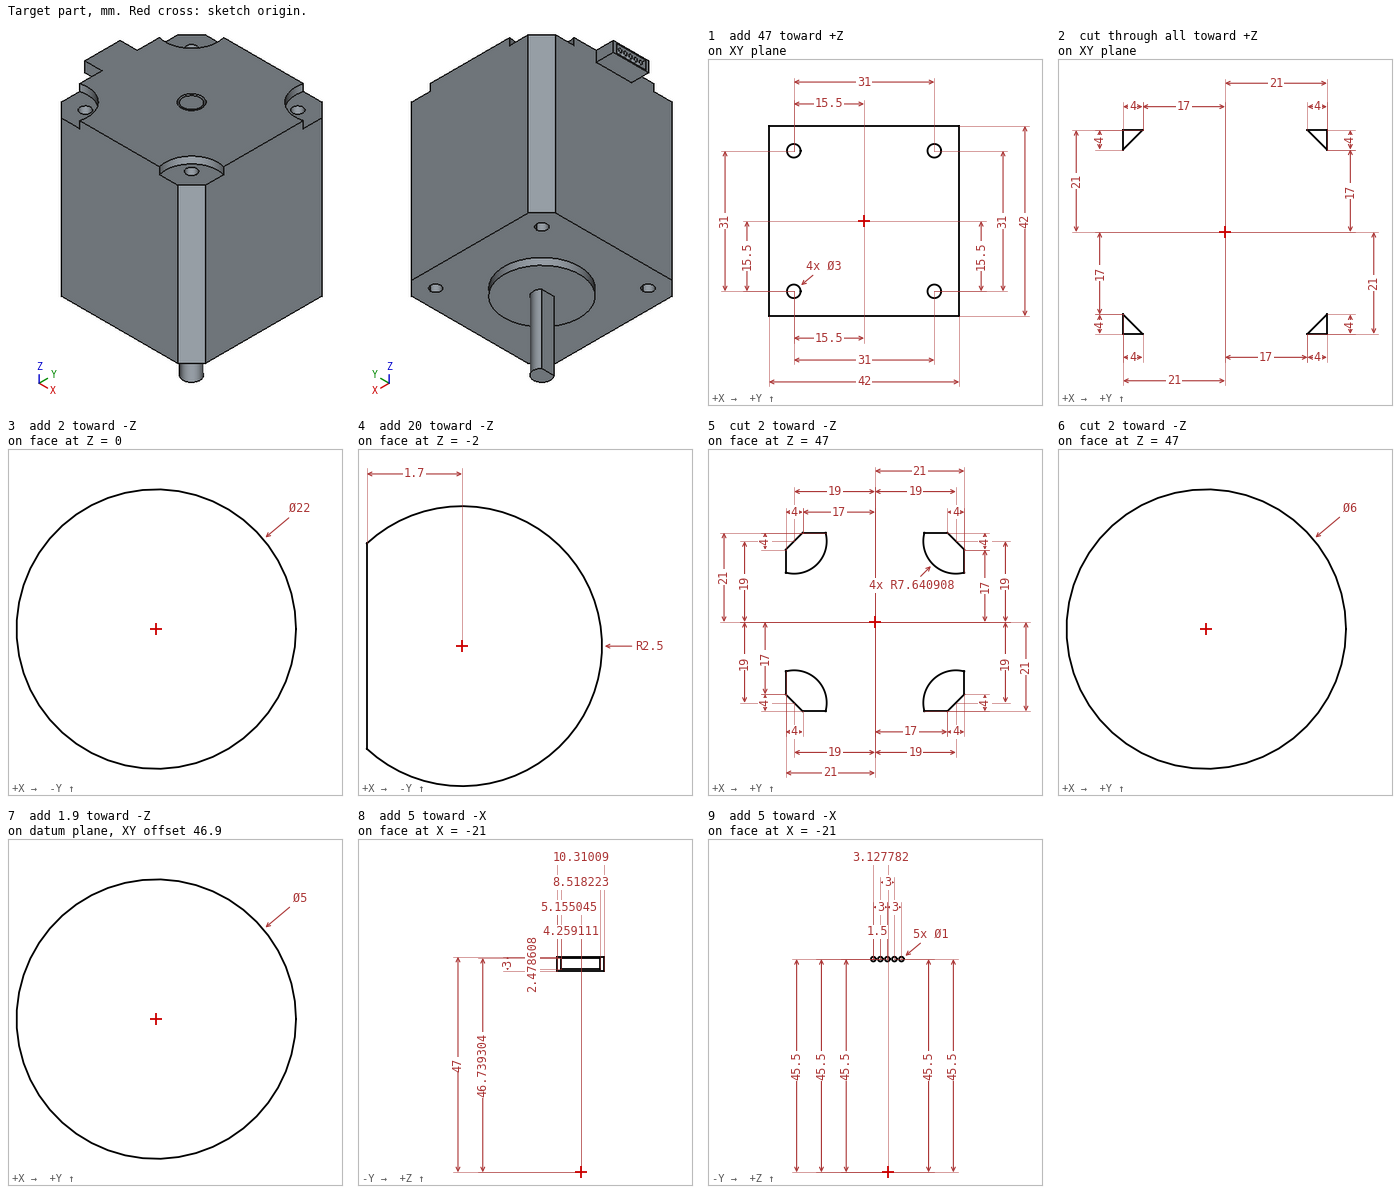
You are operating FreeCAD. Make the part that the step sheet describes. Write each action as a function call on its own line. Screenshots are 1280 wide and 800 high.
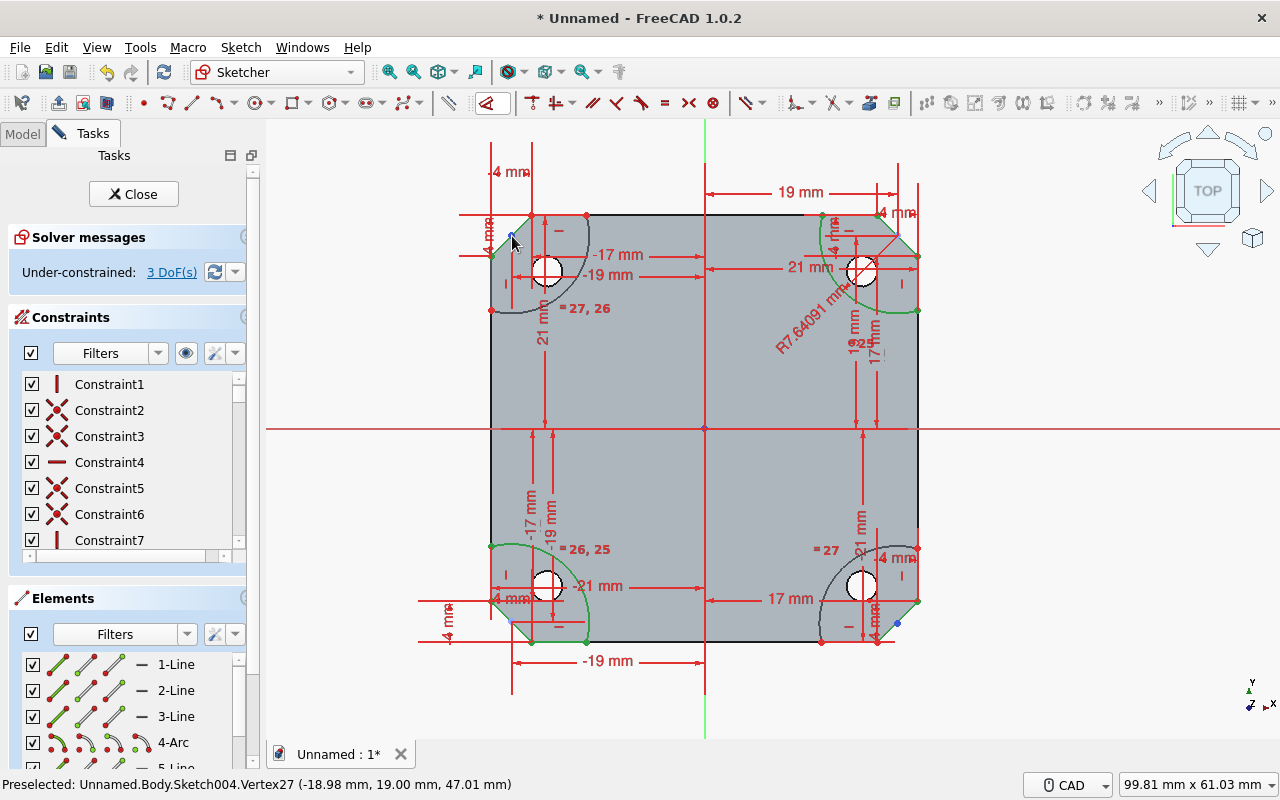
click(512, 236)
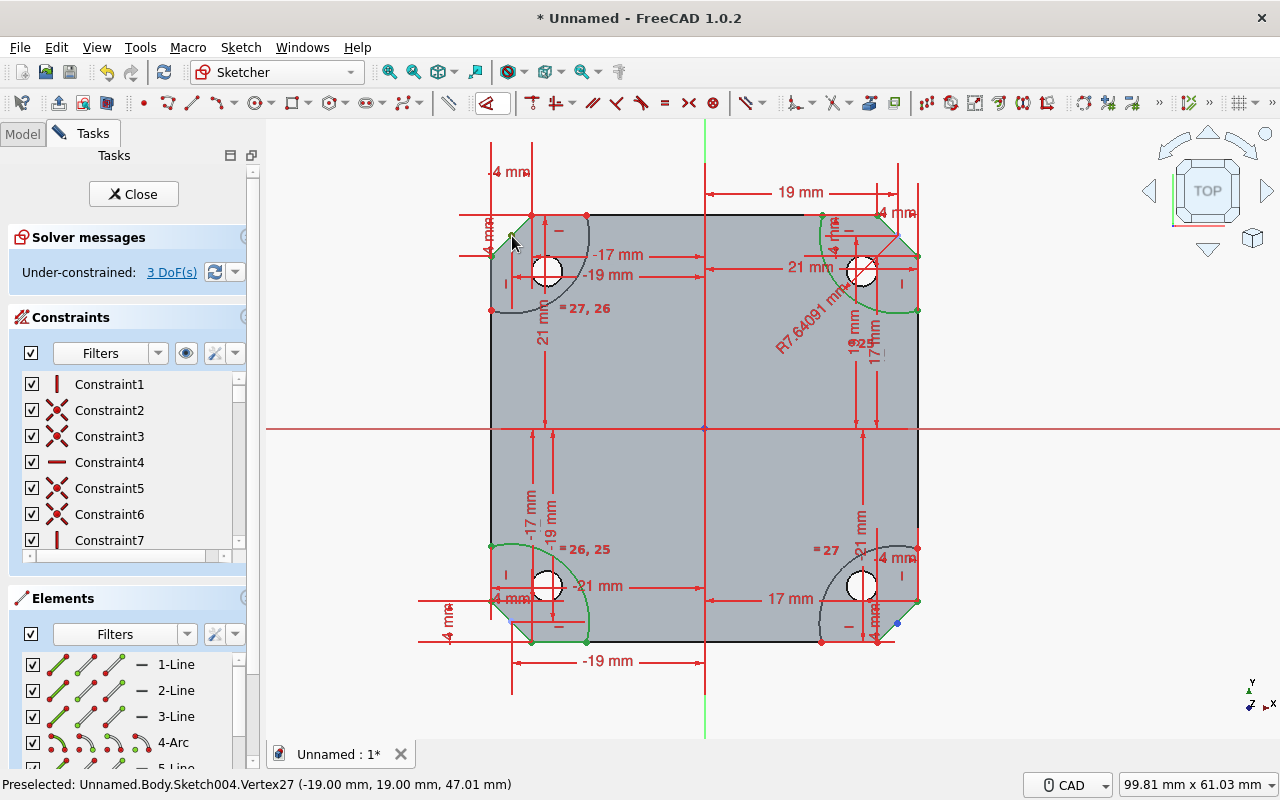
click(504, 104)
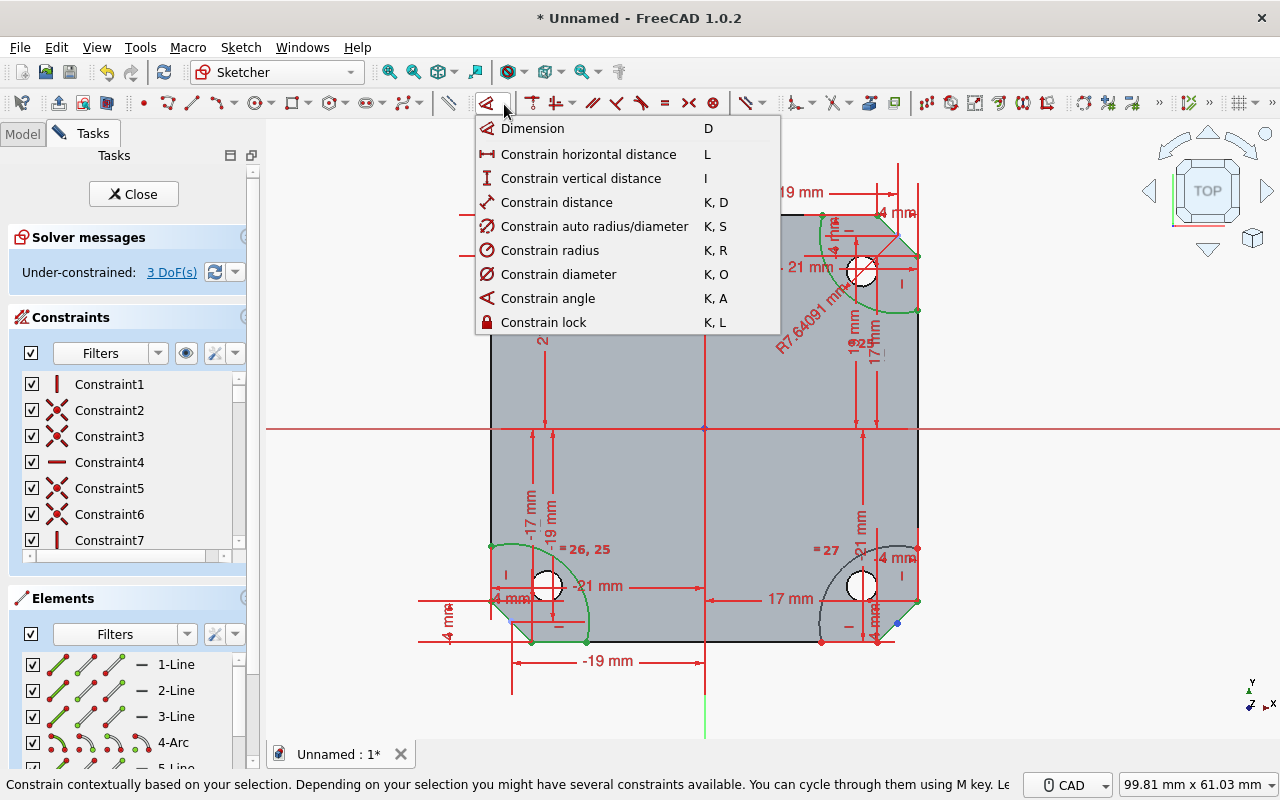
click(628, 178)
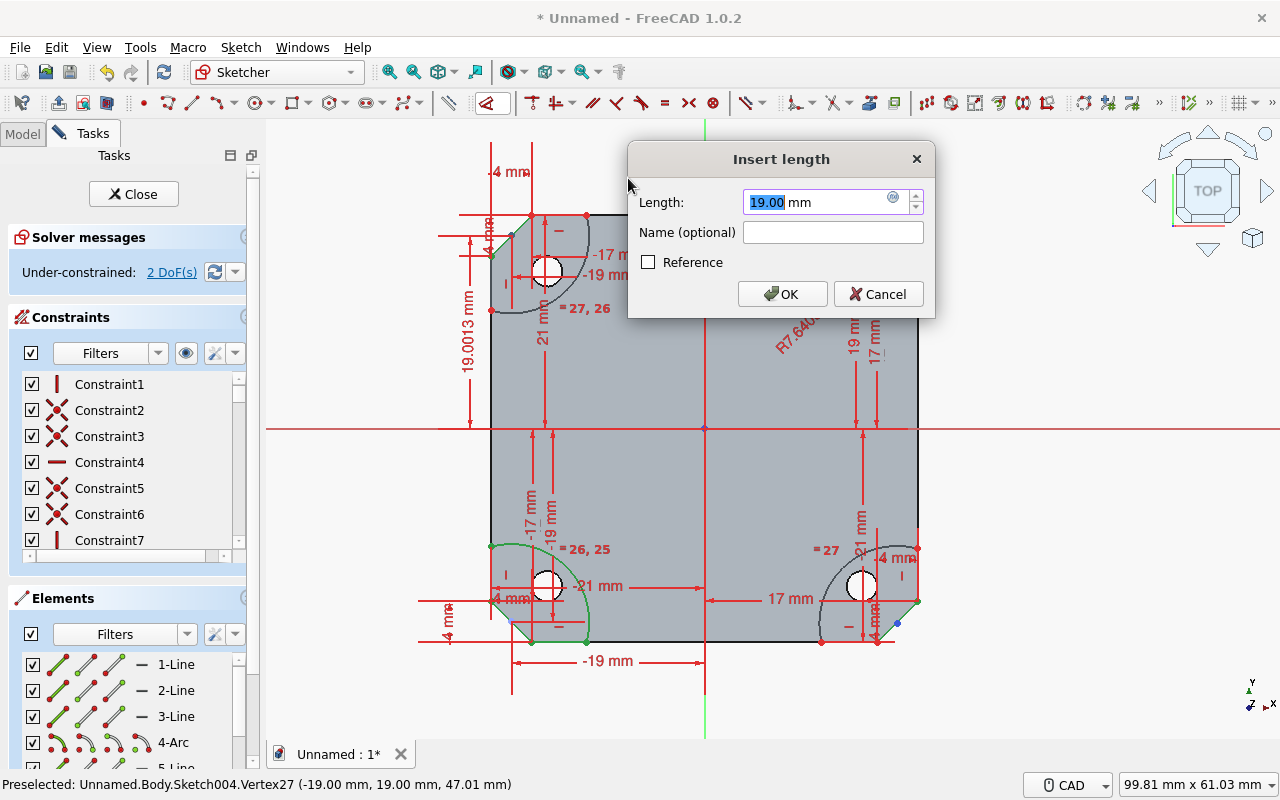
text(19)
key(Return)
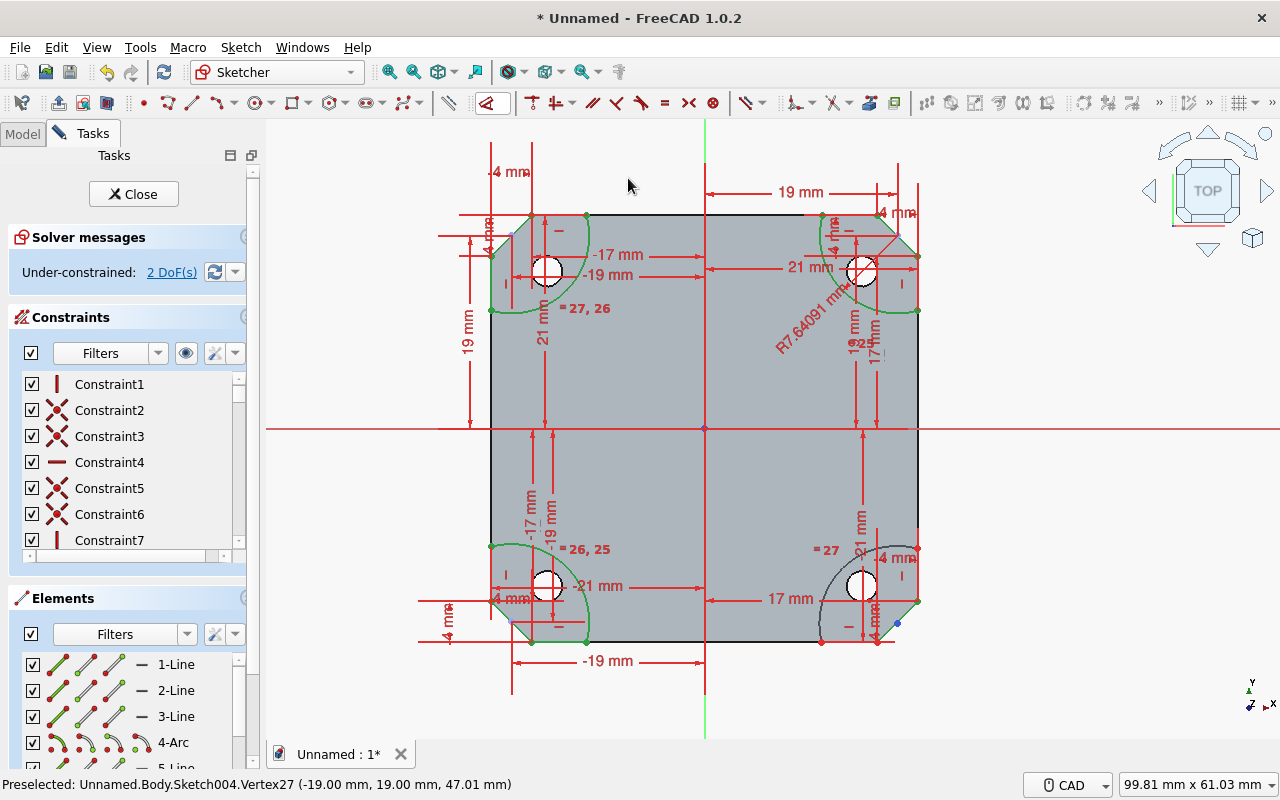
click(897, 624)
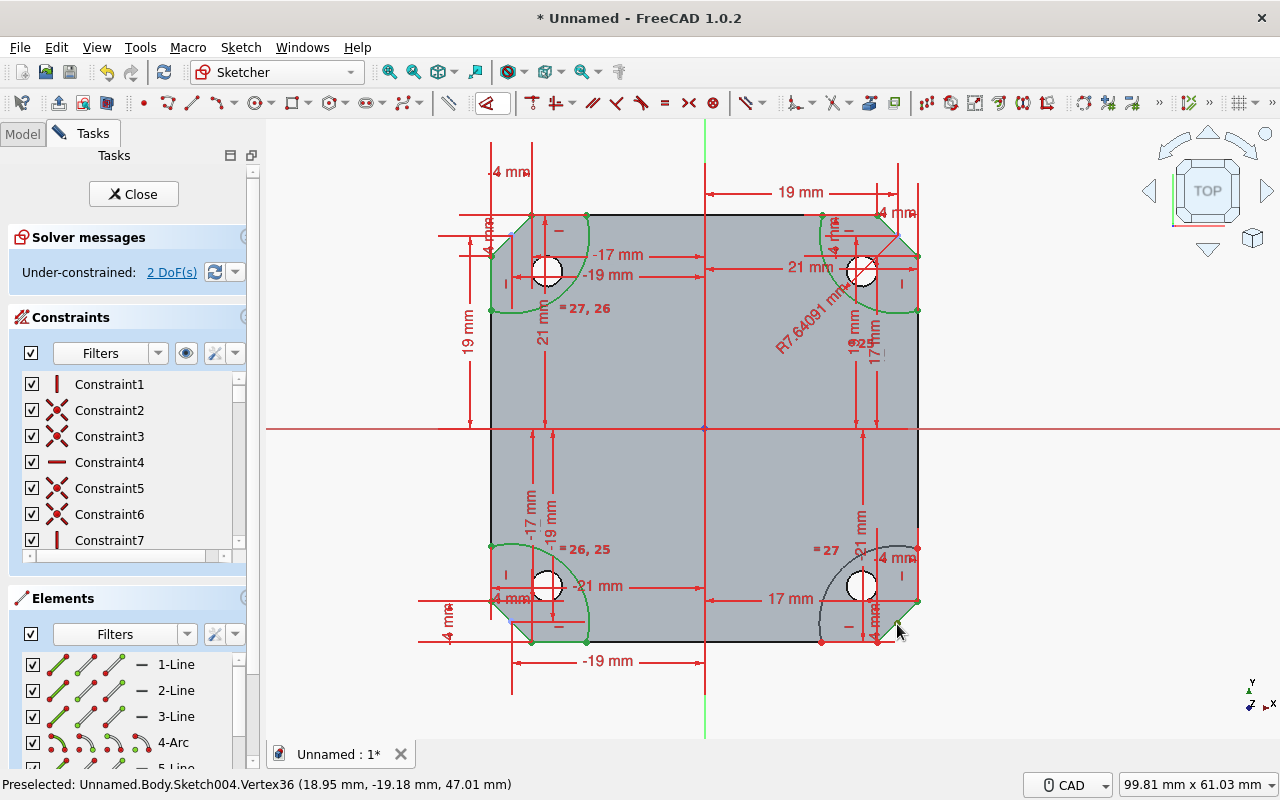
key(l)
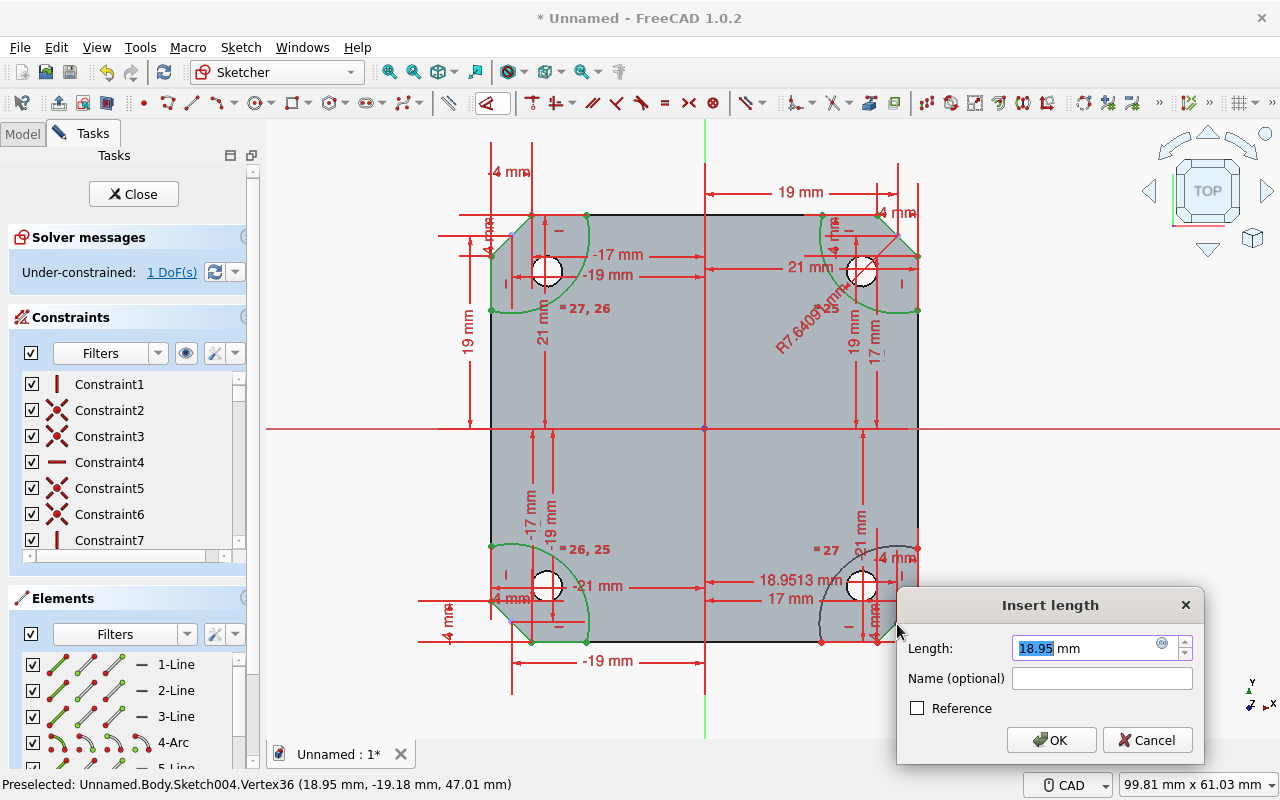
text(19)
key(Return)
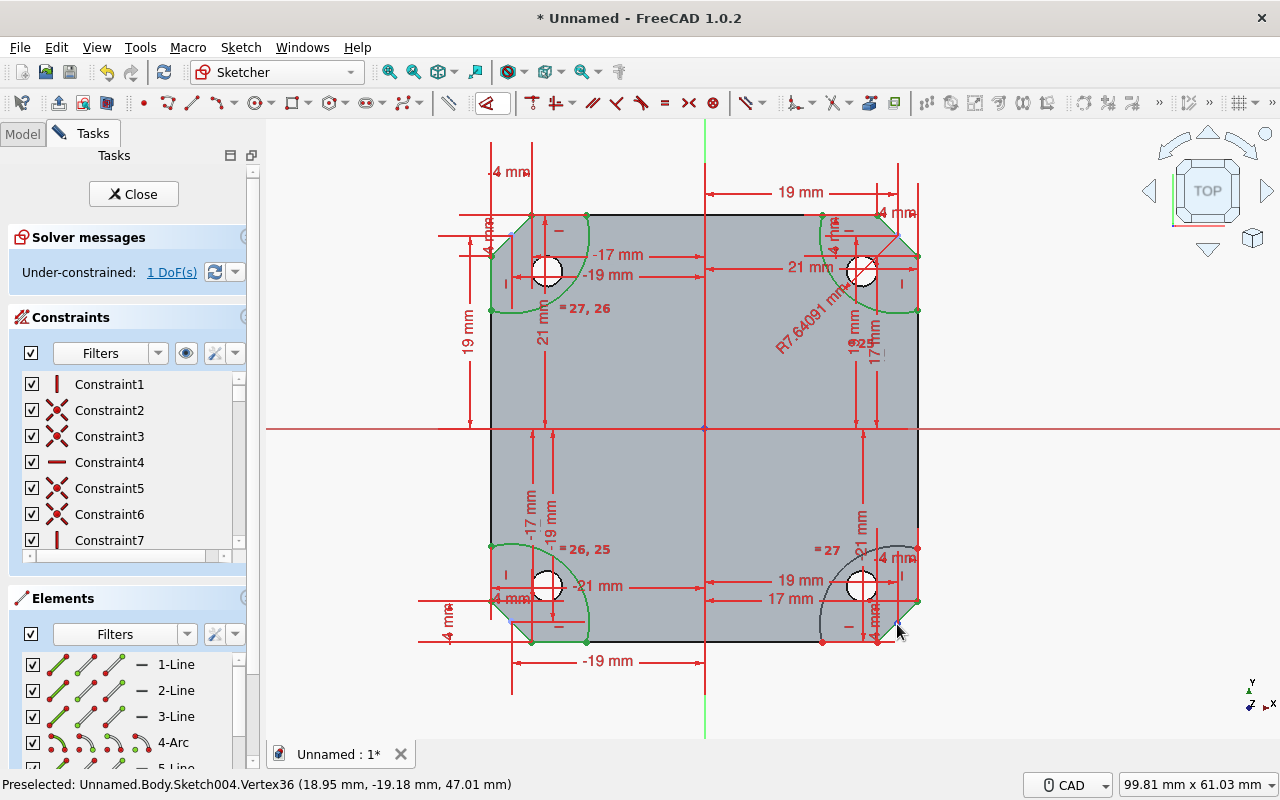
click(898, 624)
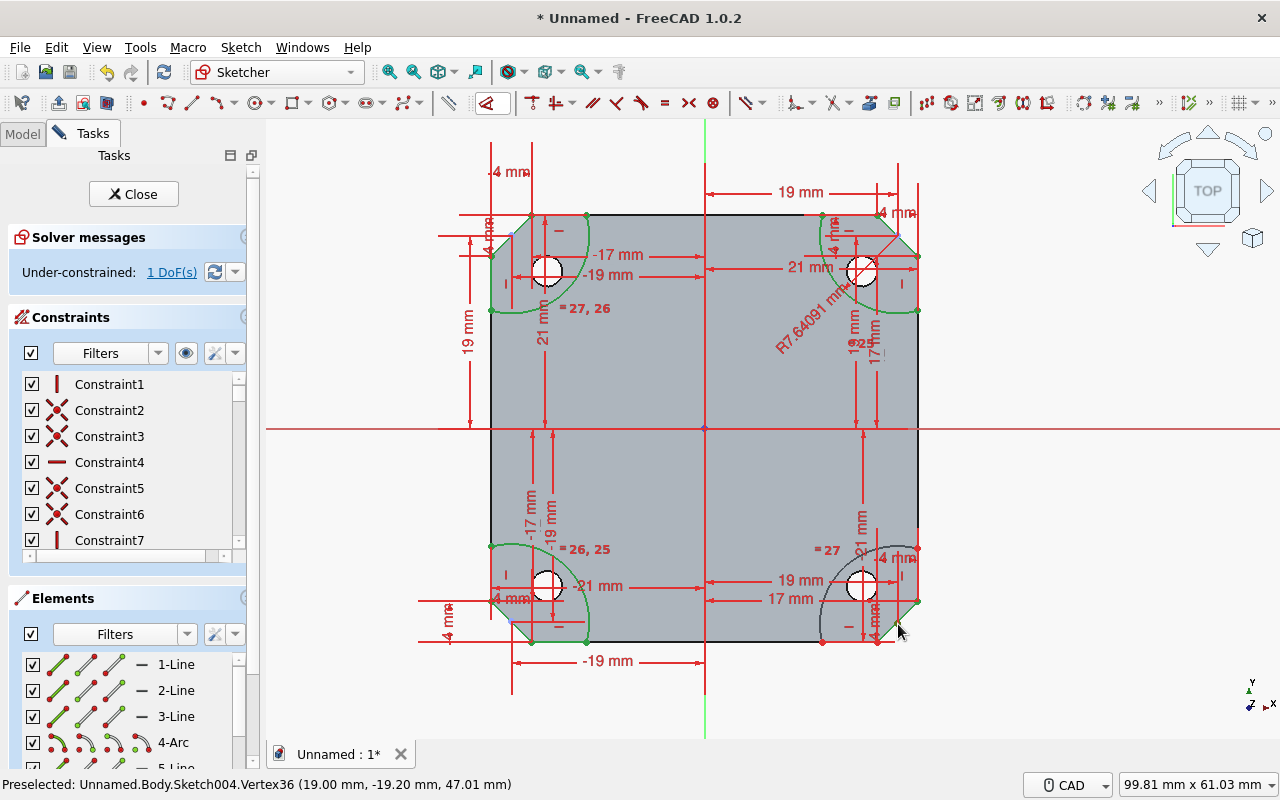
click(504, 104)